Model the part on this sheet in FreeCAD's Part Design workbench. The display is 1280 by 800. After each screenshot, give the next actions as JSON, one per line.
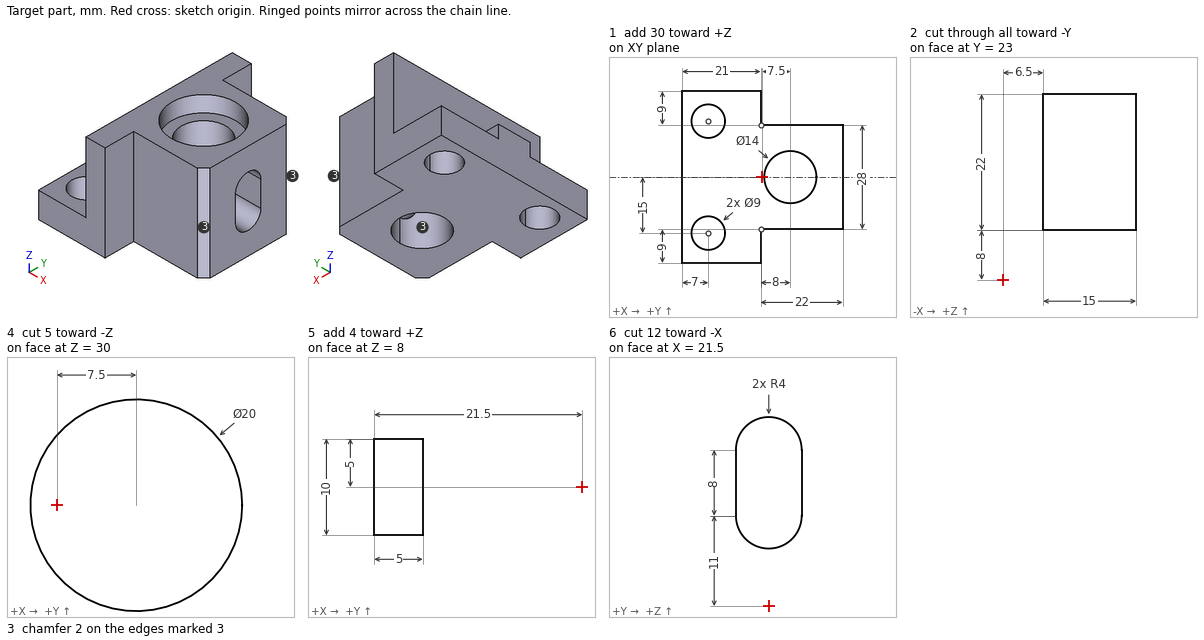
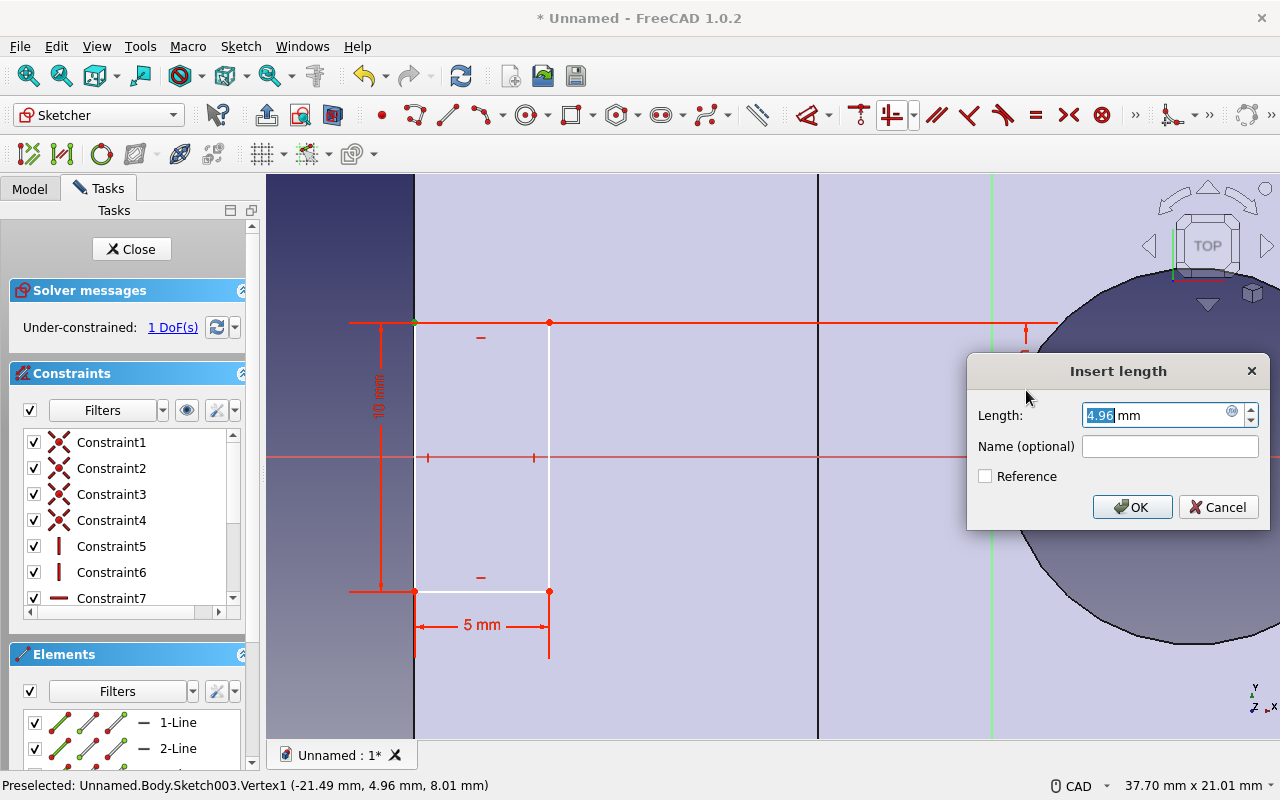
{"action": "type", "text": "5"}
{"action": "key", "text": "Return"}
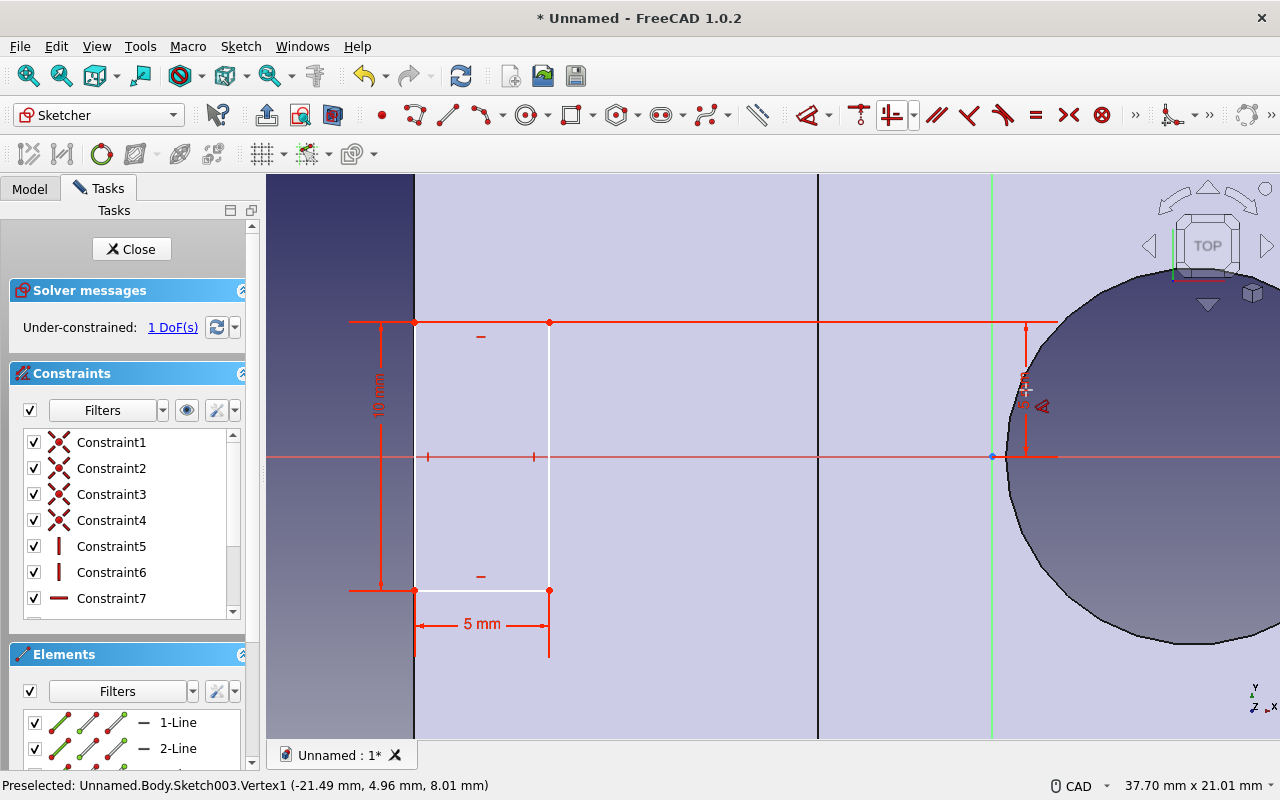
{"action": "left_click", "coordinate": [415, 322]}
{"action": "left_click", "coordinate": [703, 288]}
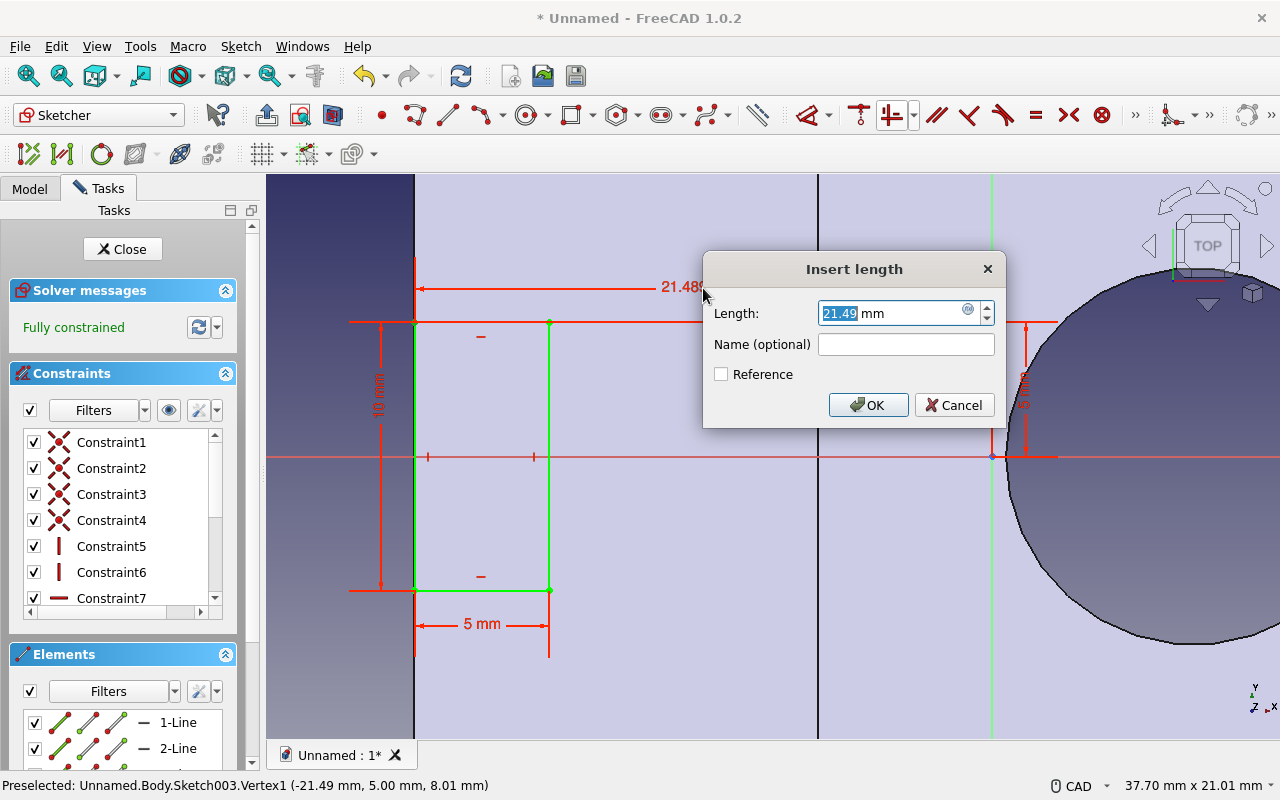
{"action": "type", "text": "21.5"}
{"action": "key", "text": "Return"}
{"action": "key", "text": "Escape"}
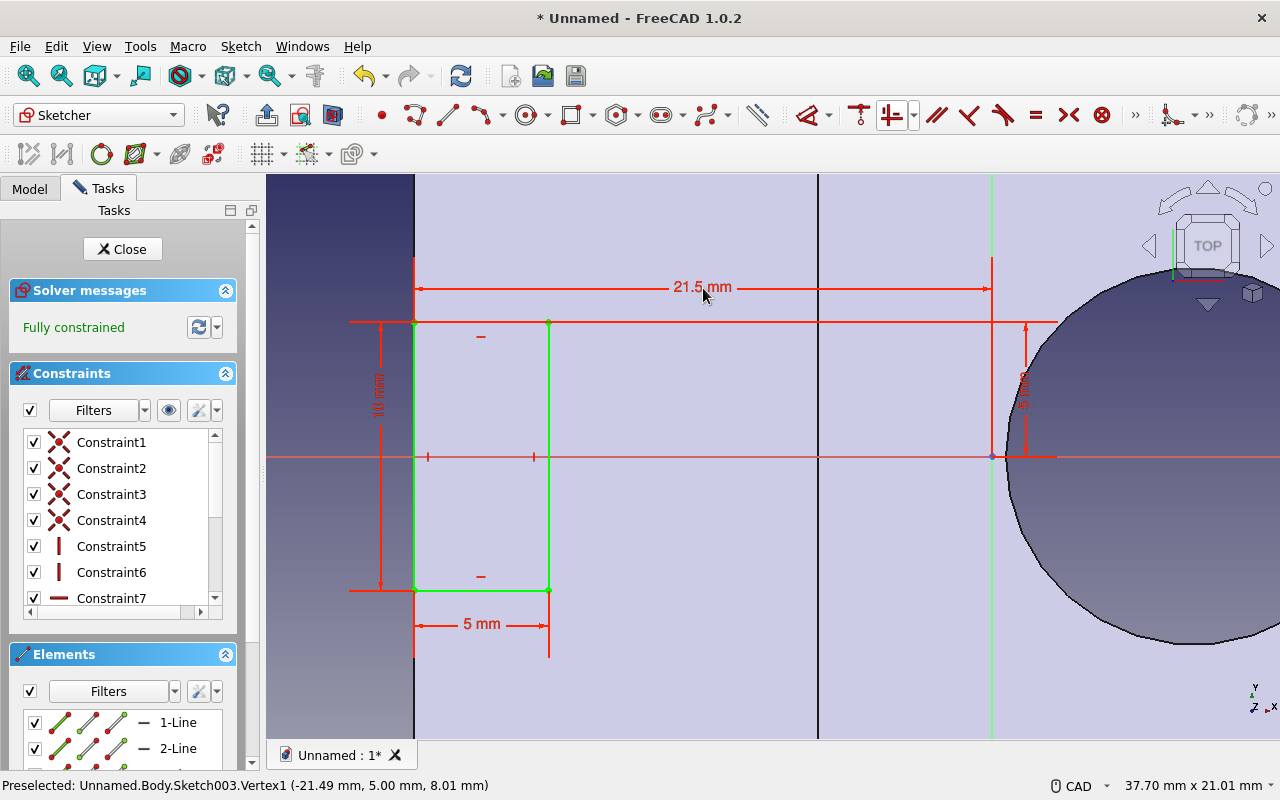
{"action": "left_click", "coordinate": [123, 249]}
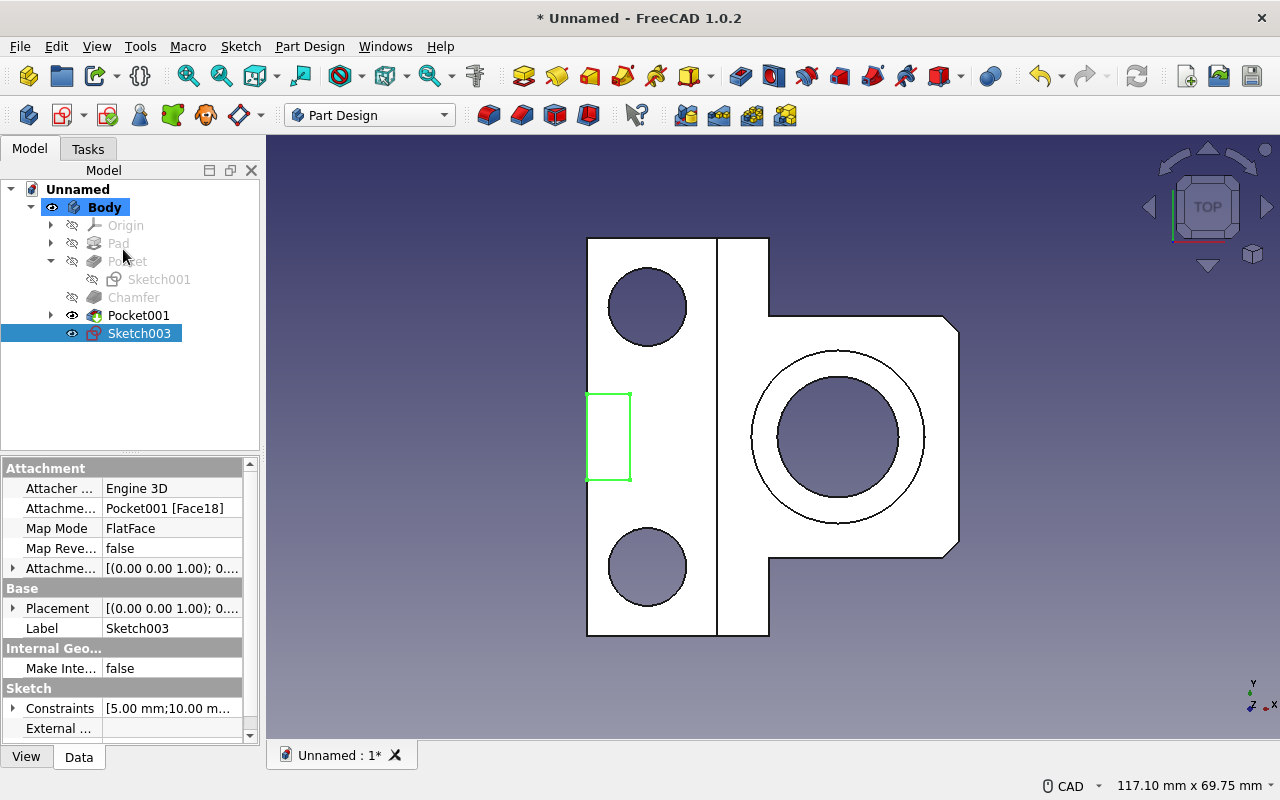
{"action": "left_click", "coordinate": [524, 76]}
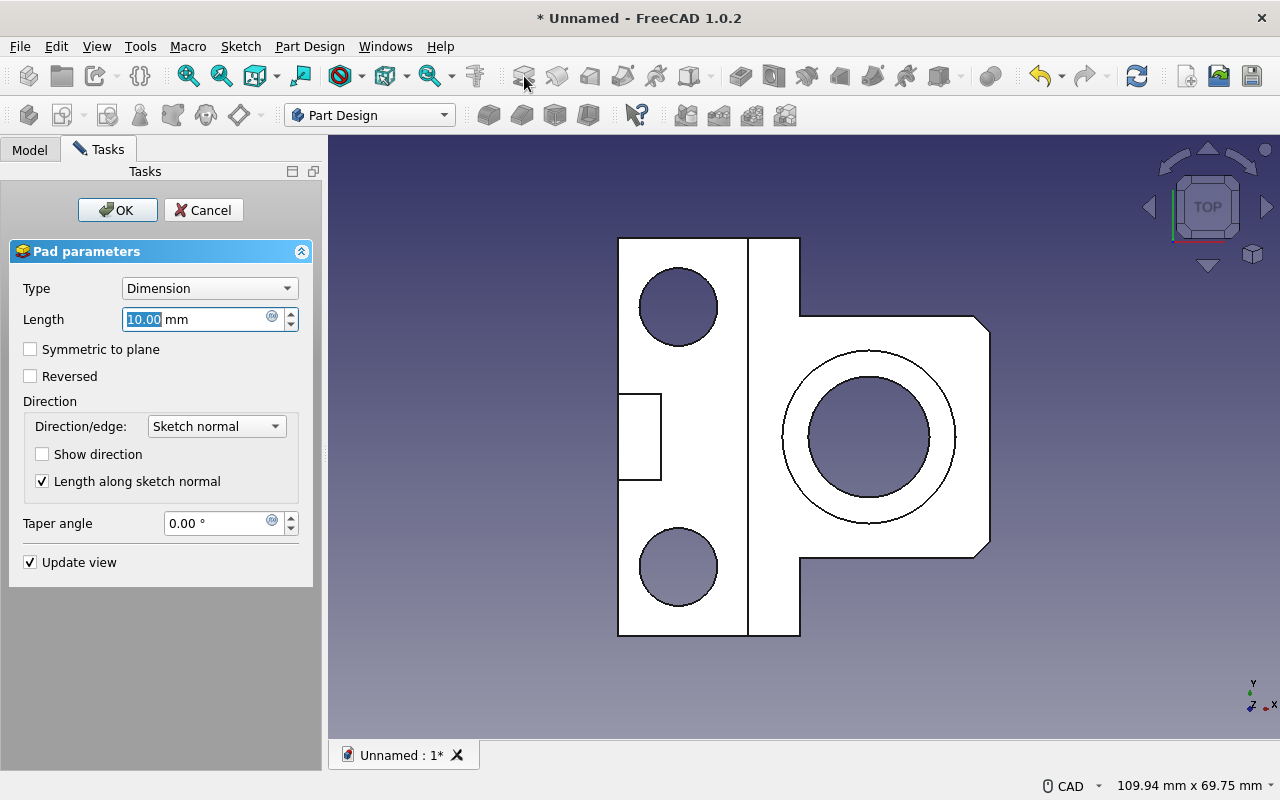
{"action": "type", "text": "4"}
{"action": "key", "text": "Tab"}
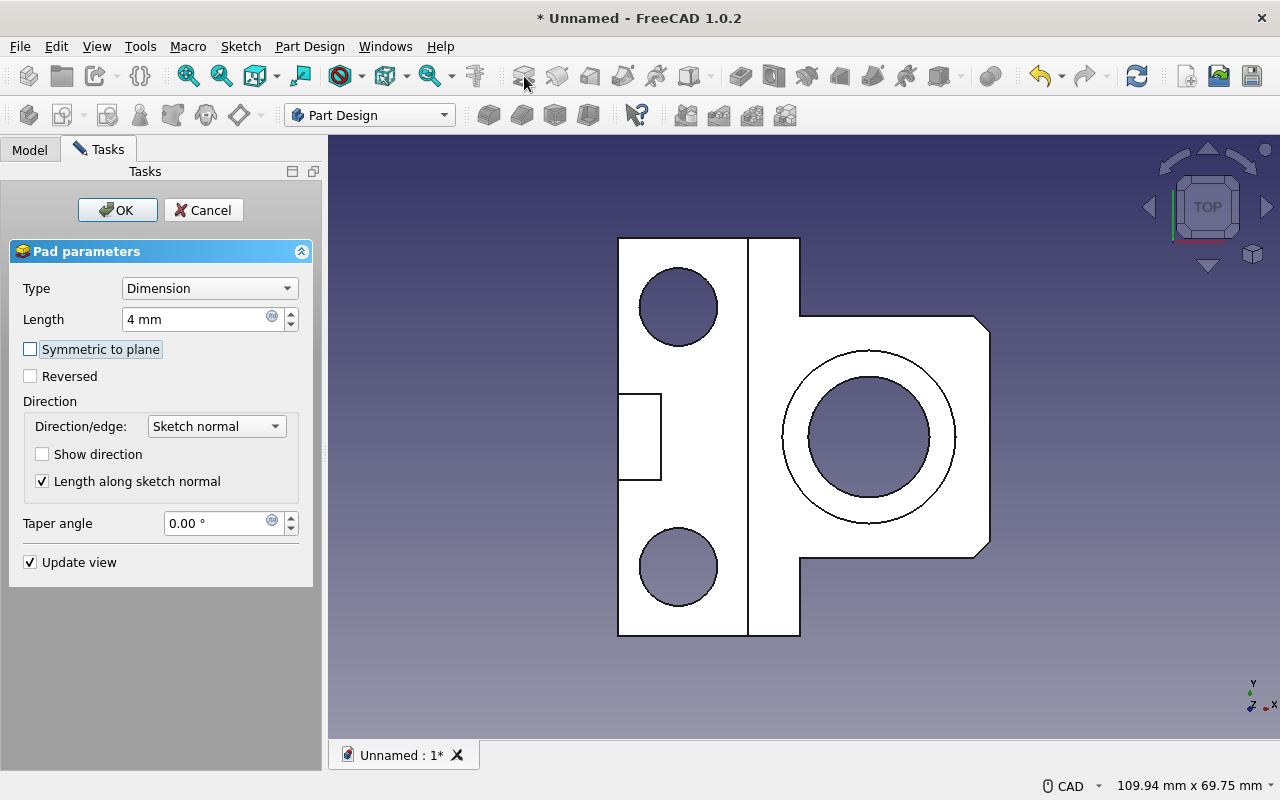
{"action": "left_click", "coordinate": [118, 210]}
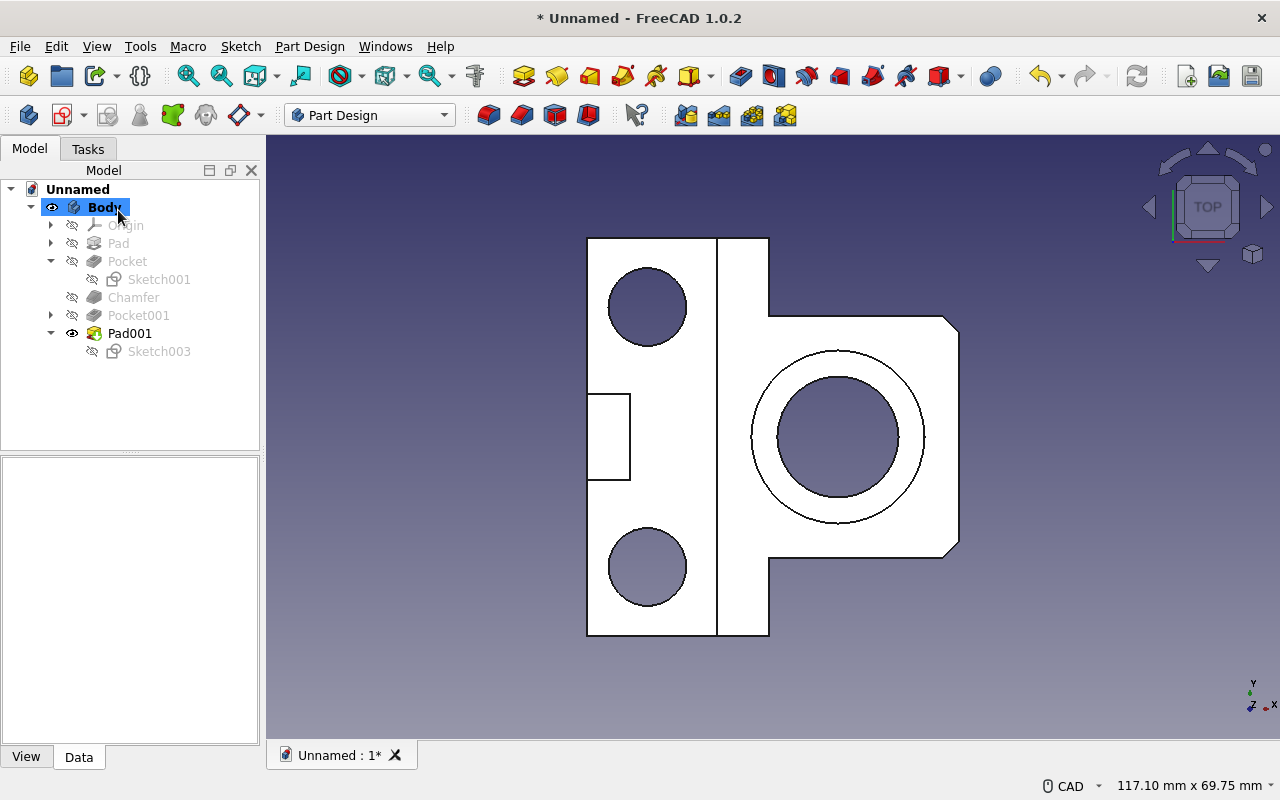
{"action": "key", "text": "0"}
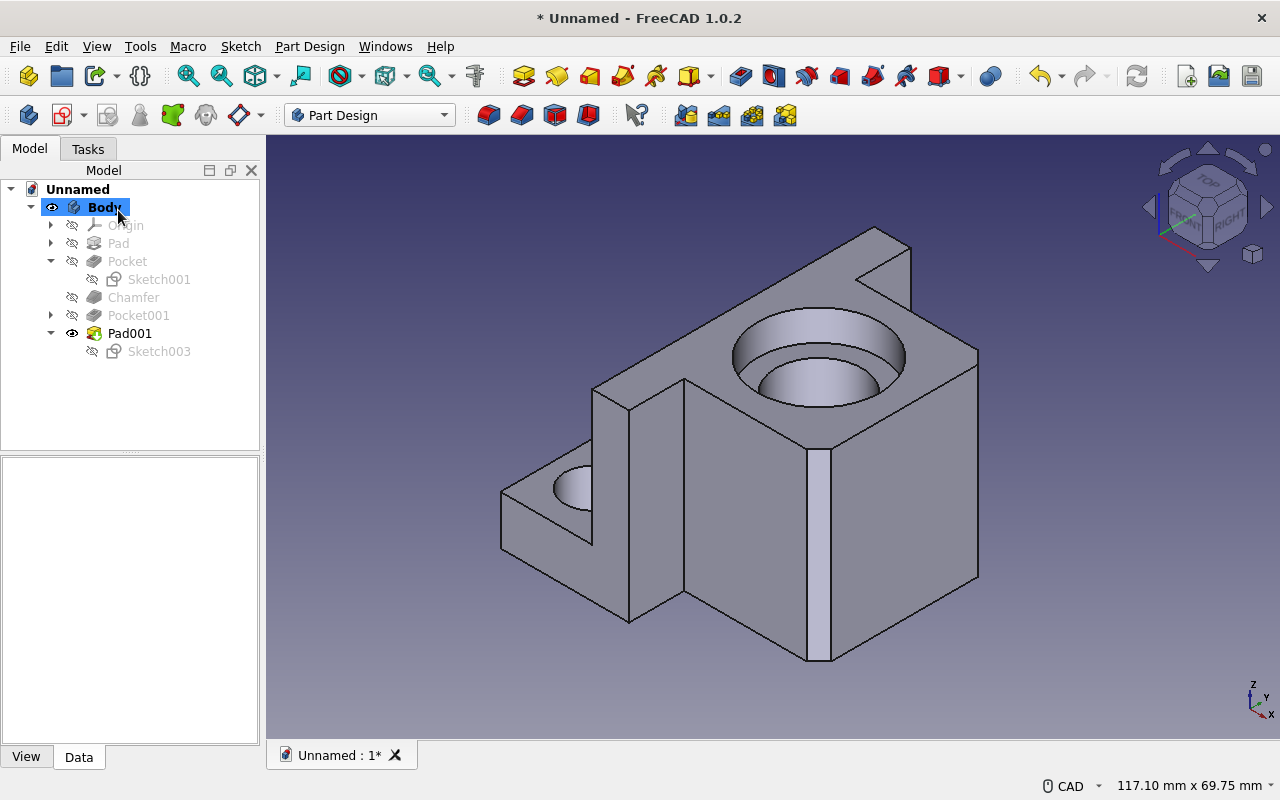
{"action": "left_click", "coordinate": [905, 512]}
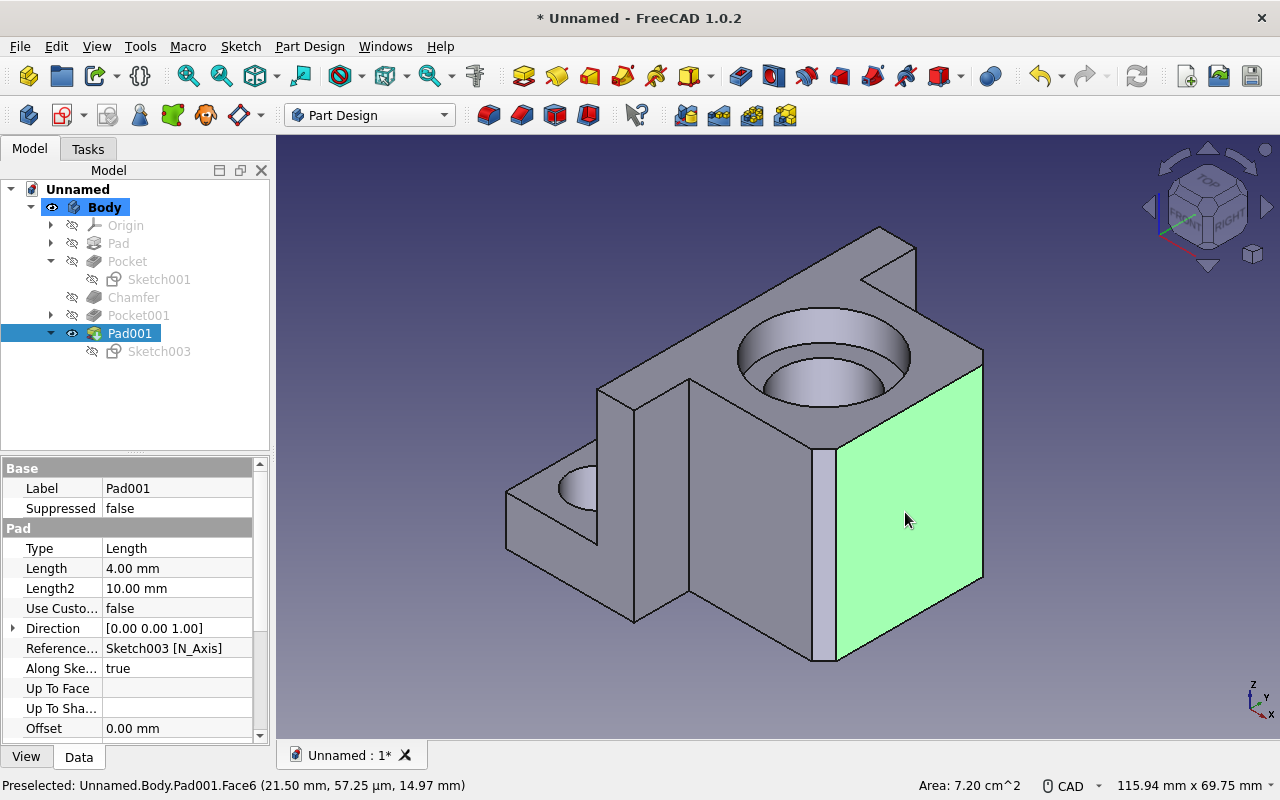
{"action": "left_click", "coordinate": [62, 116]}